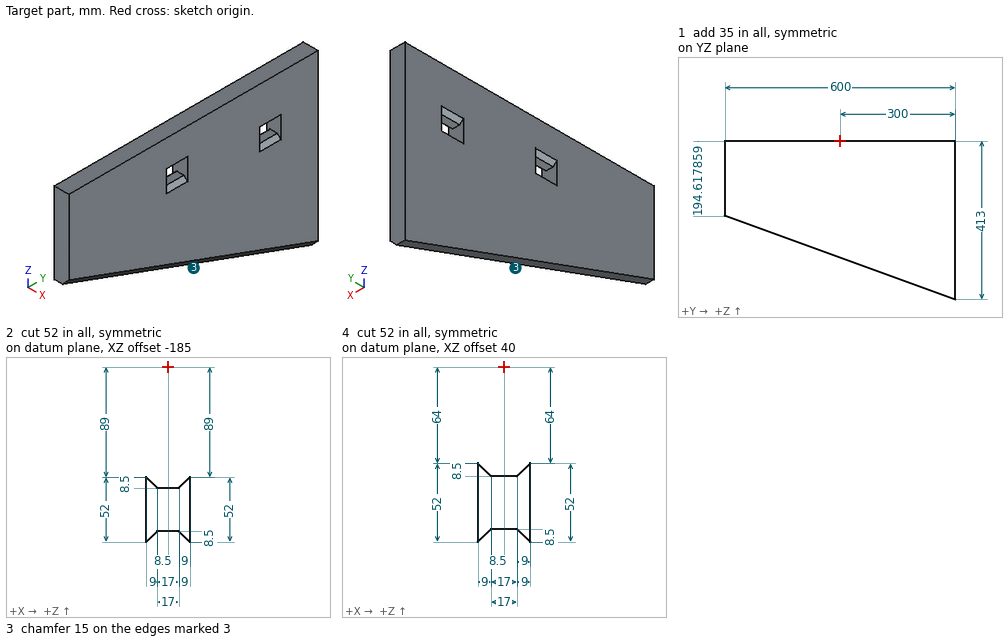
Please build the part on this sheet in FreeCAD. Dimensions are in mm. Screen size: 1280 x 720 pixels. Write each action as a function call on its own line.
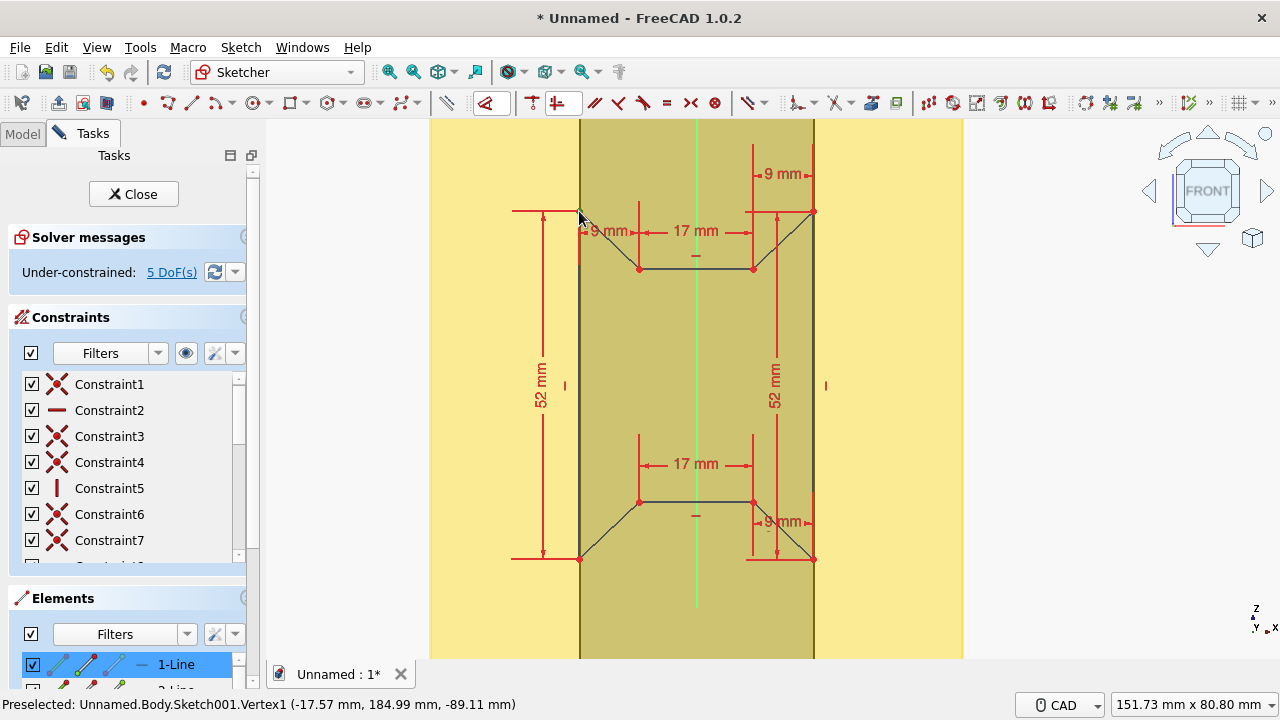
key(i)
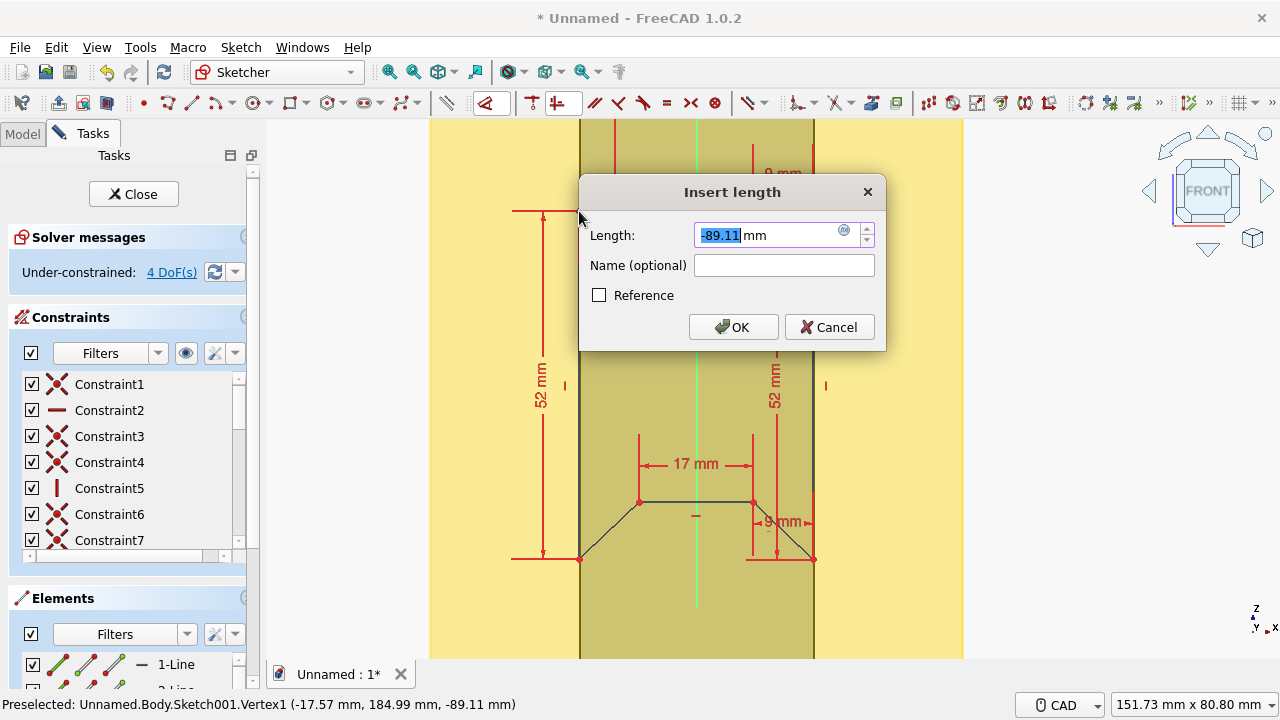
text(-89)
key(Return)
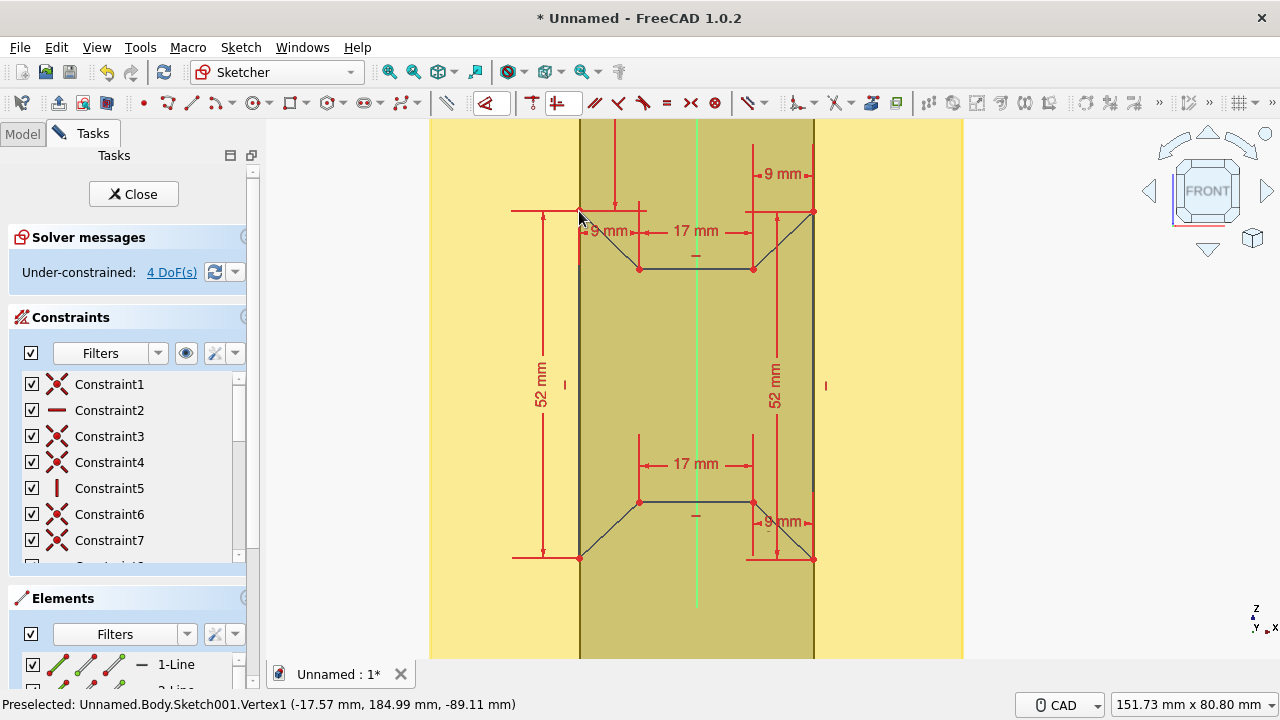
click(813, 212)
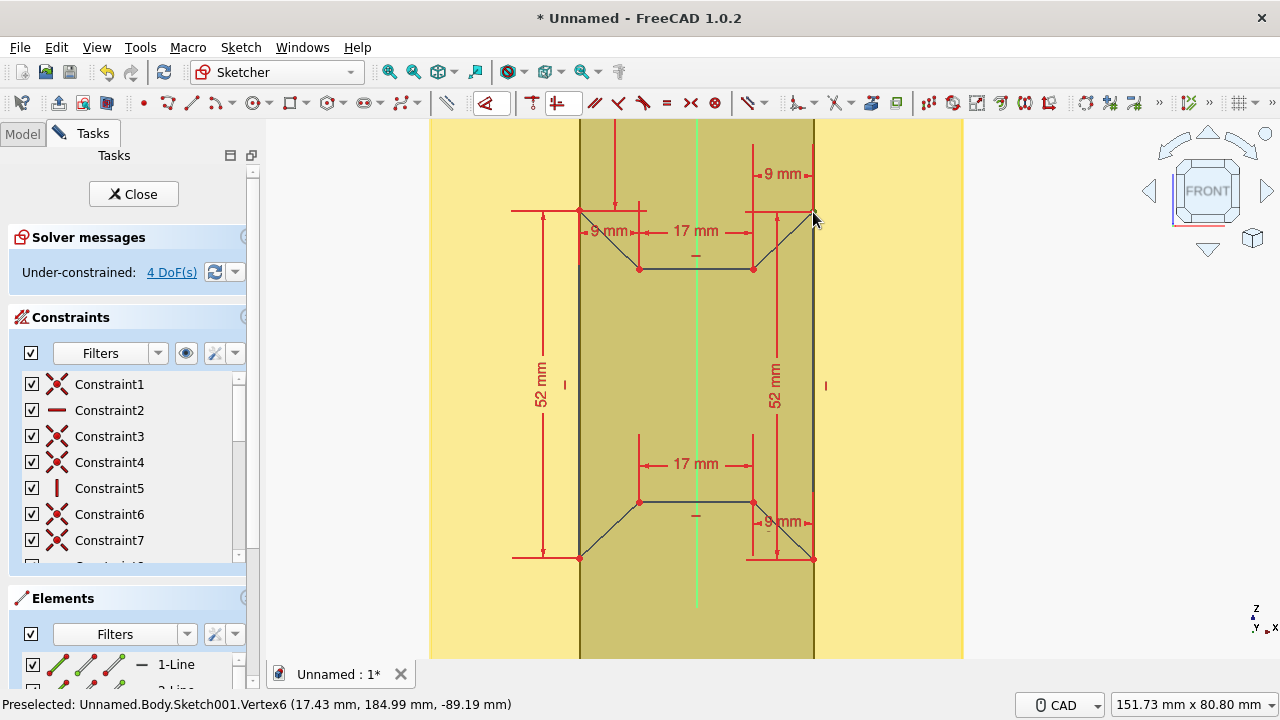
key(i)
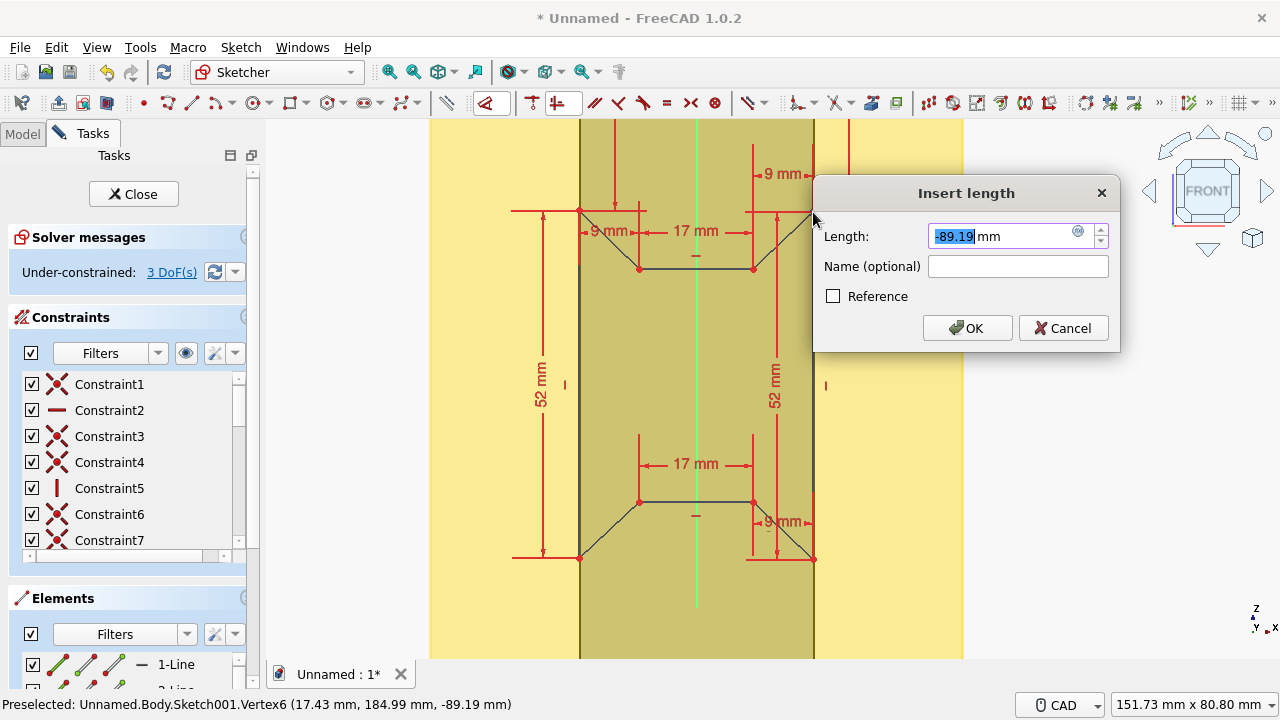
text(-89)
key(Return)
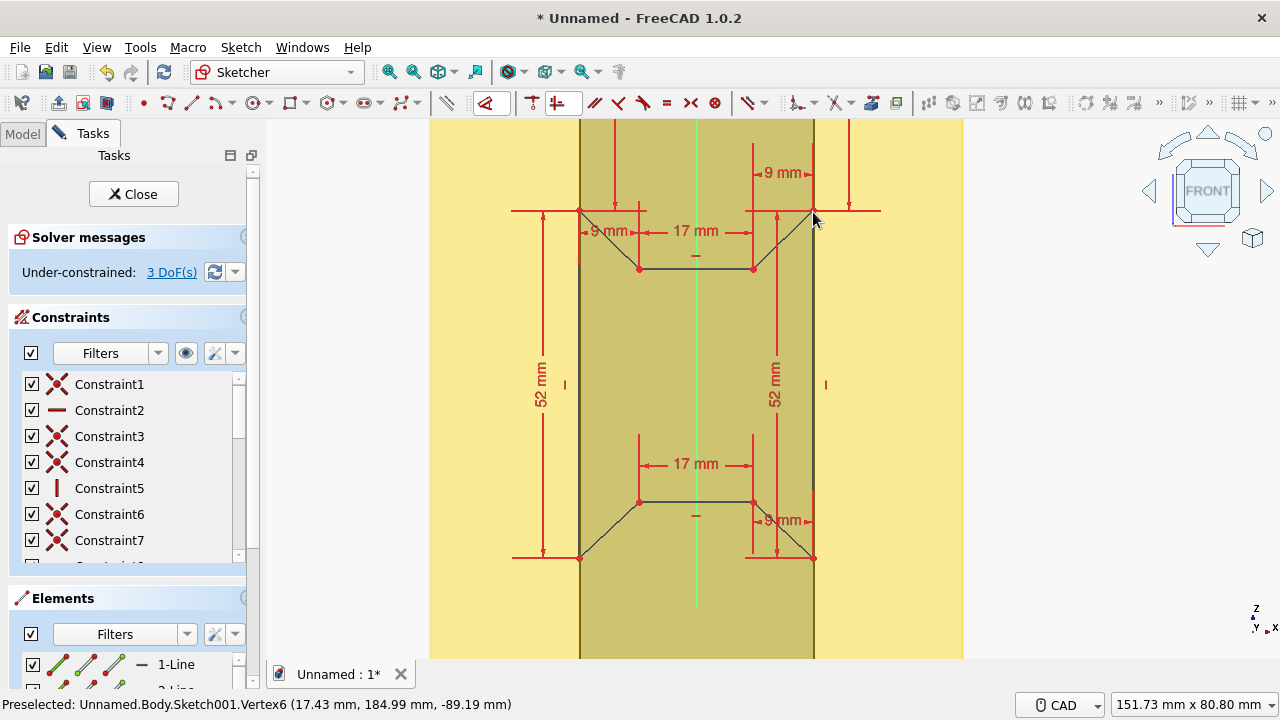
click(639, 269)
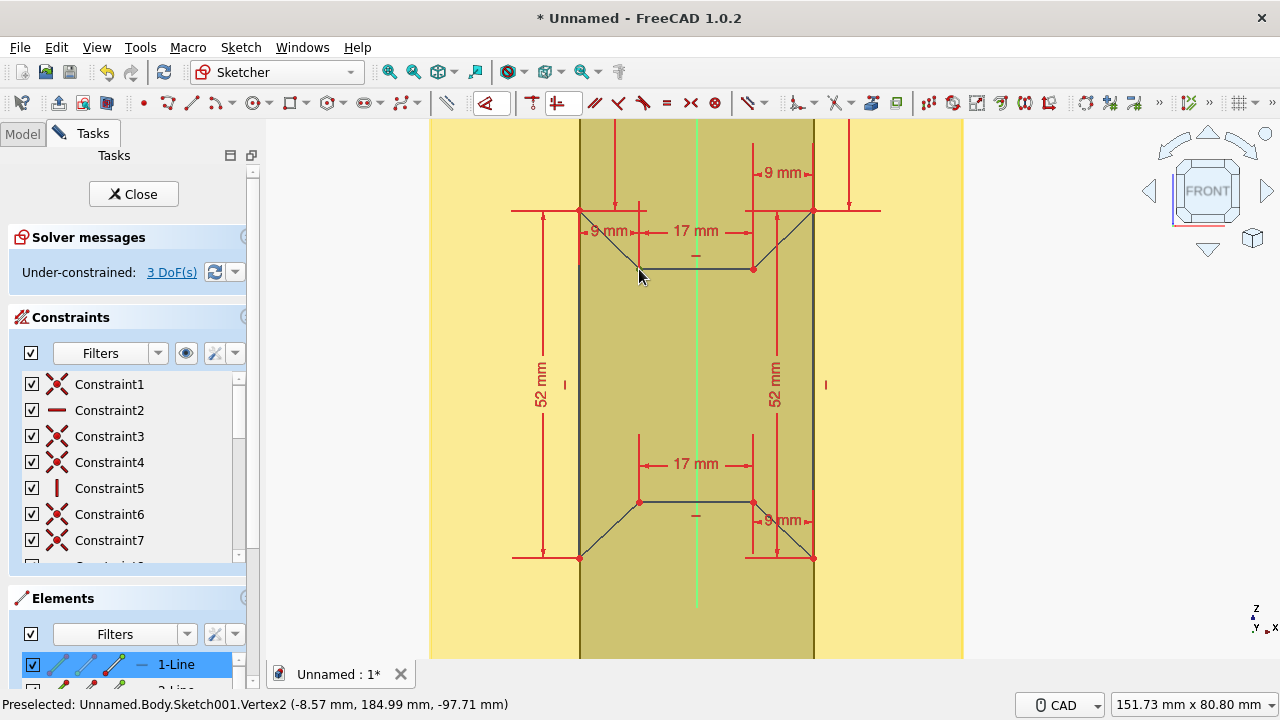
key(l)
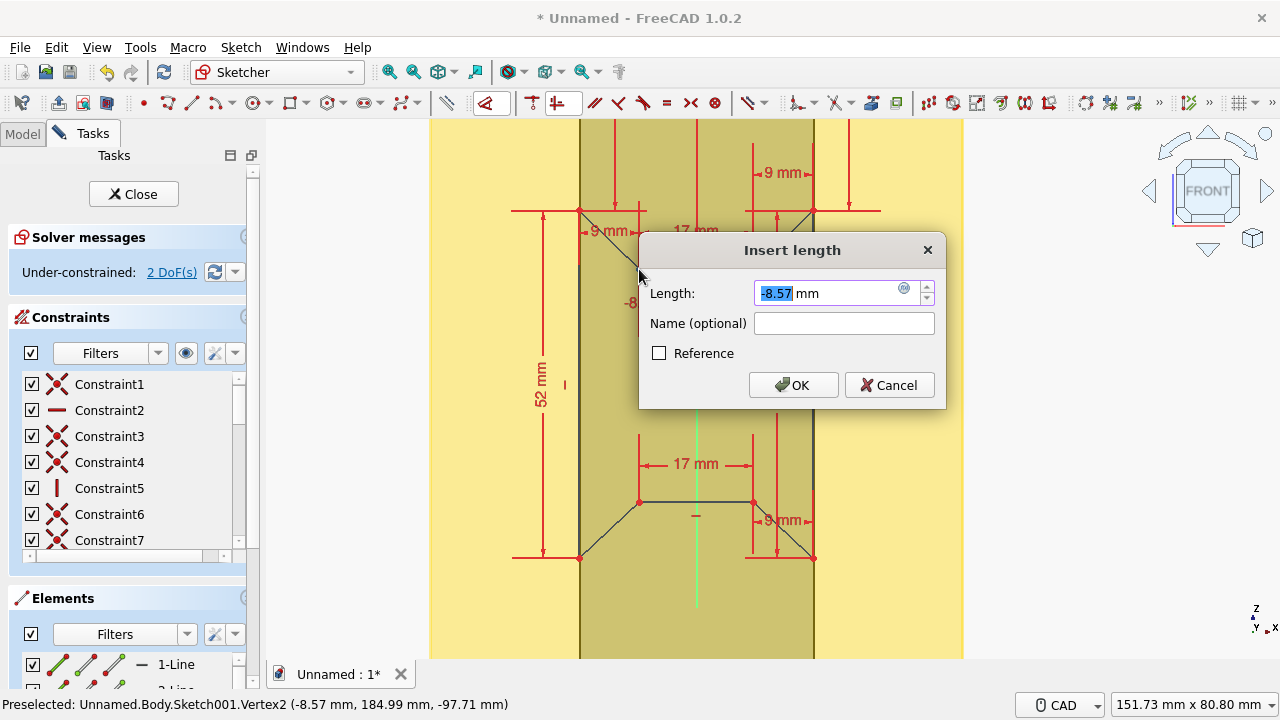
text(-8.5)
key(Return)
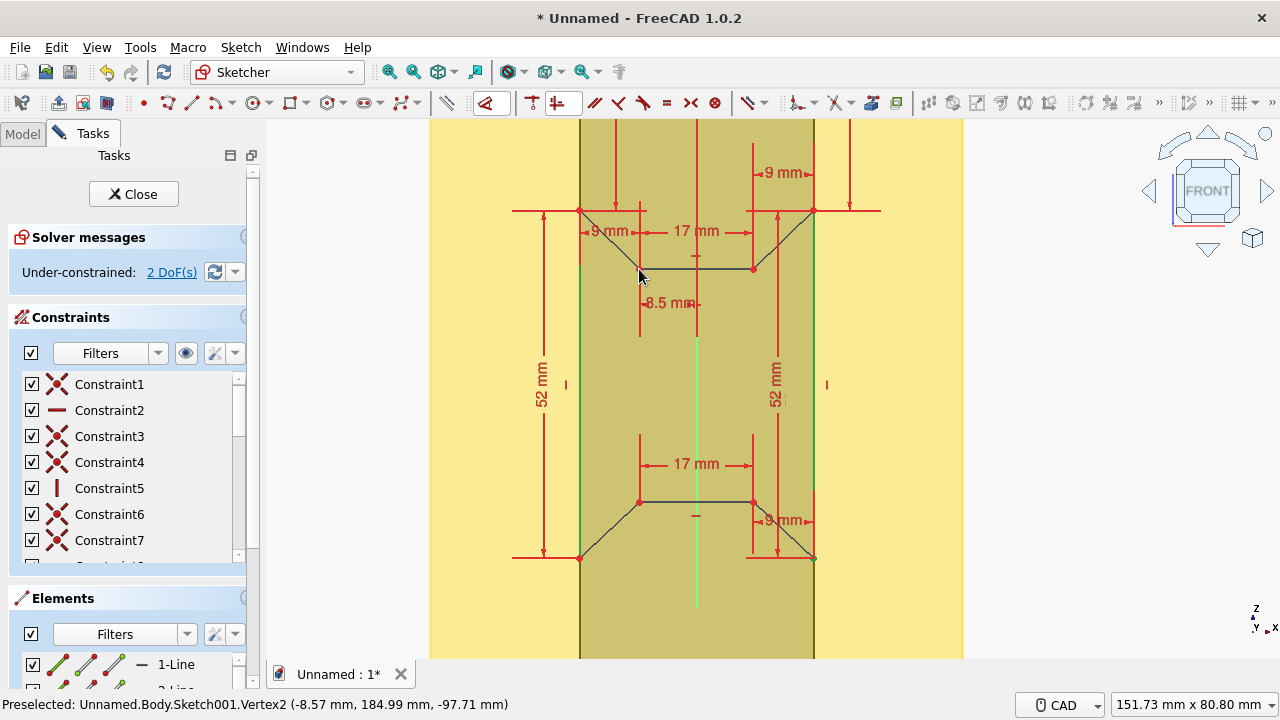
click(622, 252)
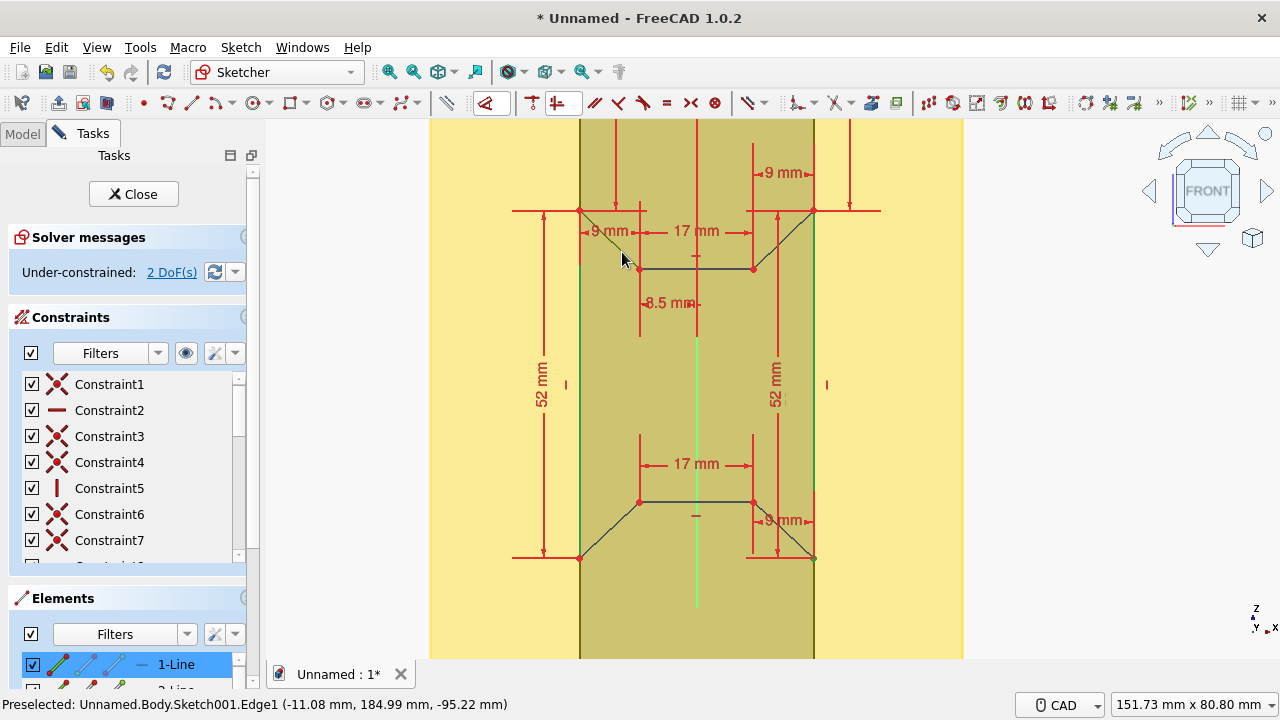
key(i)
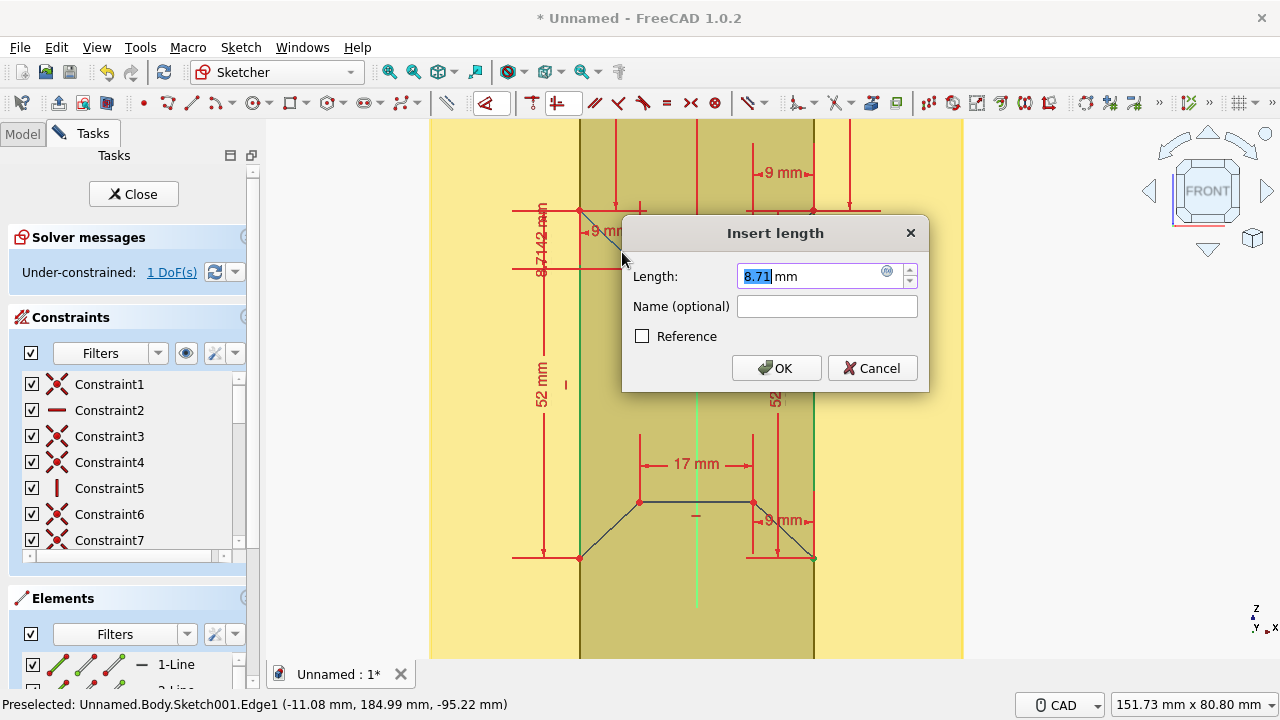
text(8.5)
key(Return)